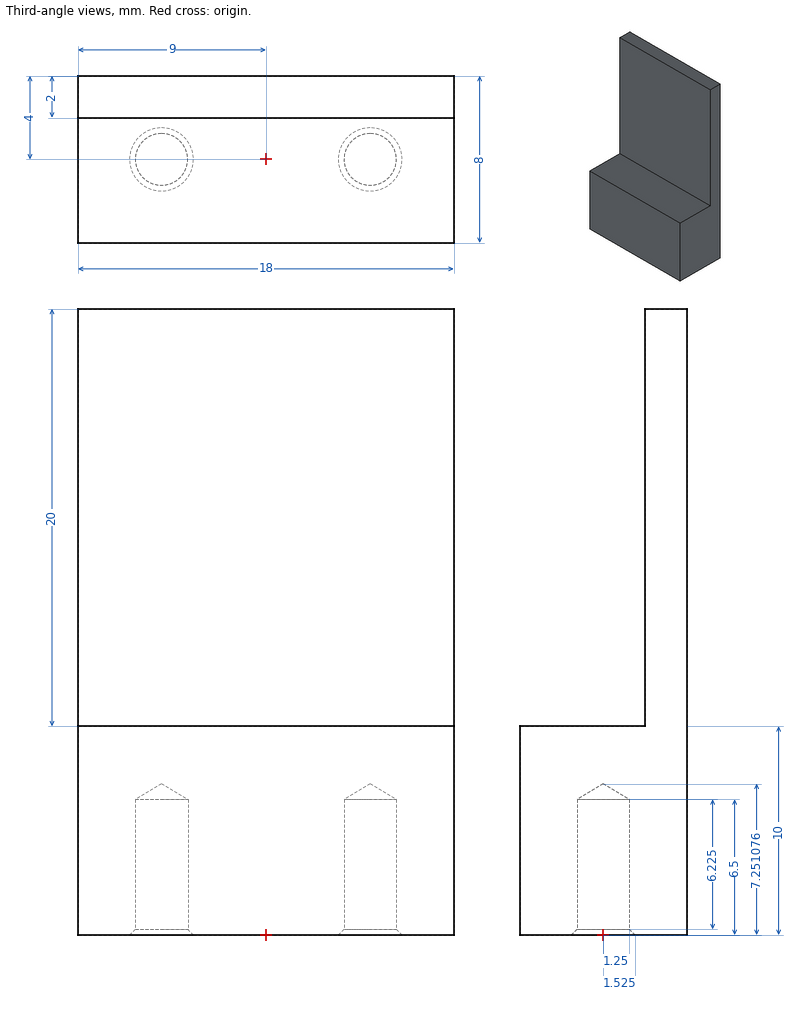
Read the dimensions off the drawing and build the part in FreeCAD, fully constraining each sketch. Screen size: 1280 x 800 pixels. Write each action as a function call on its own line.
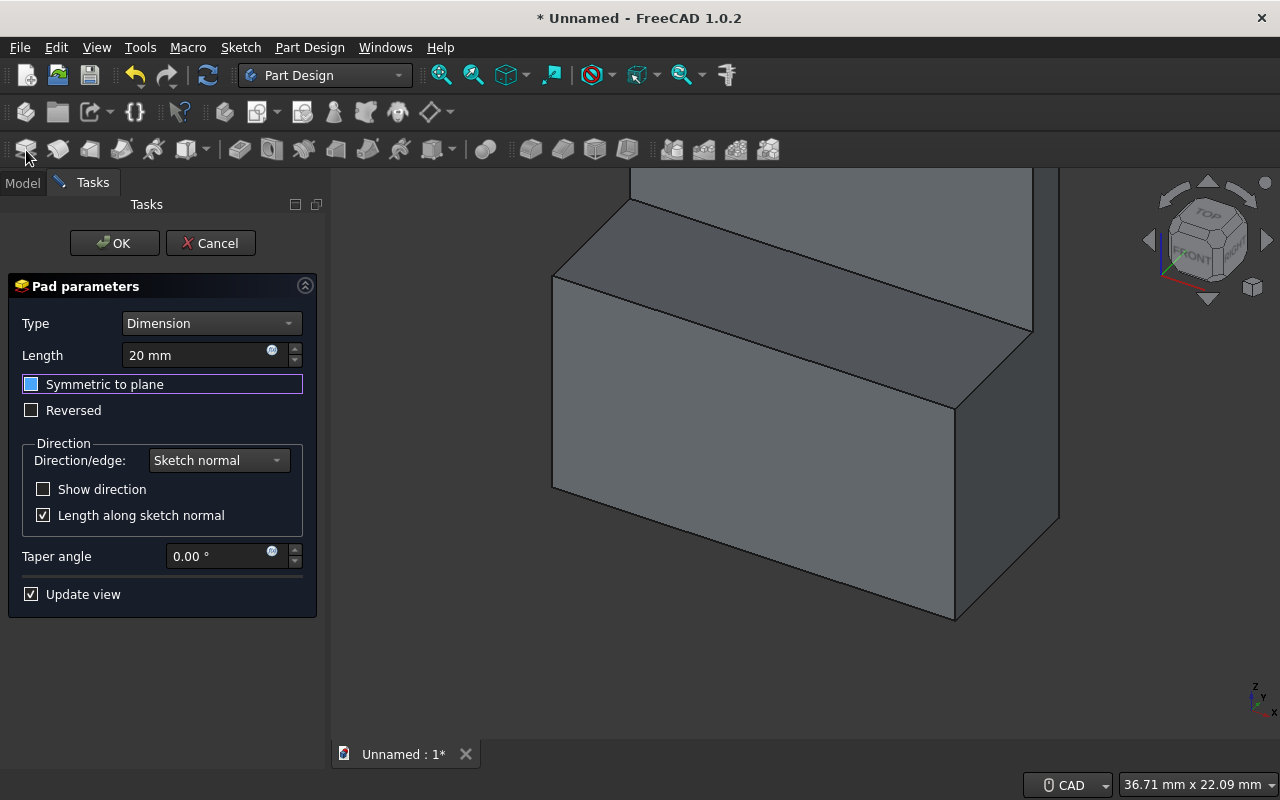
click(115, 243)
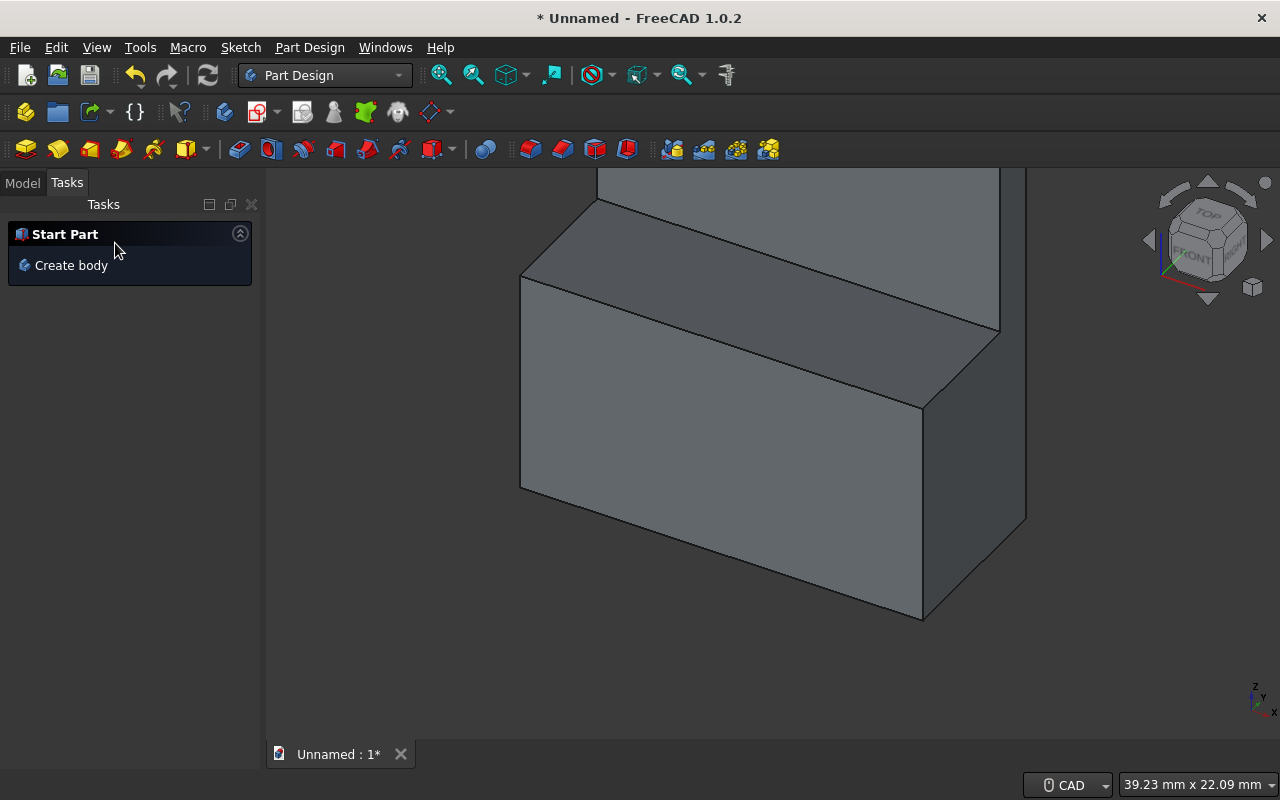
click(442, 76)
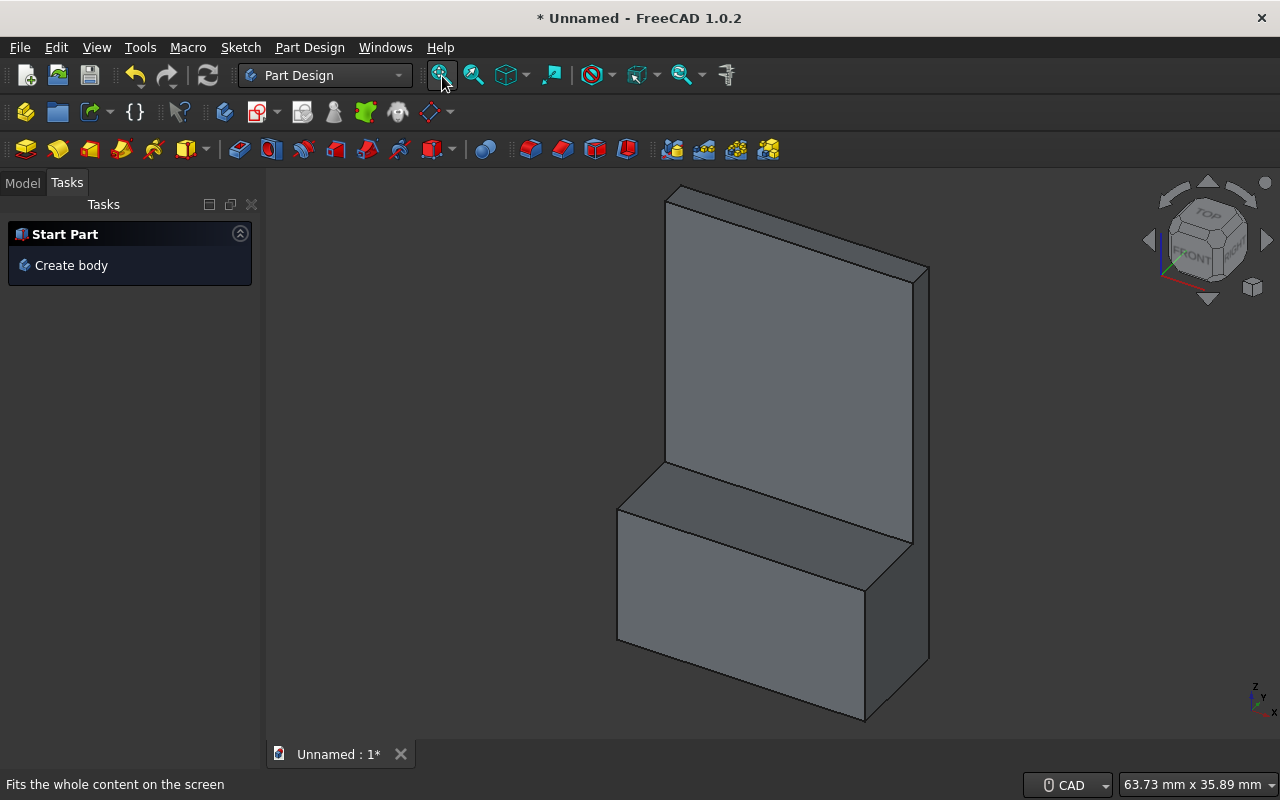
click(23, 182)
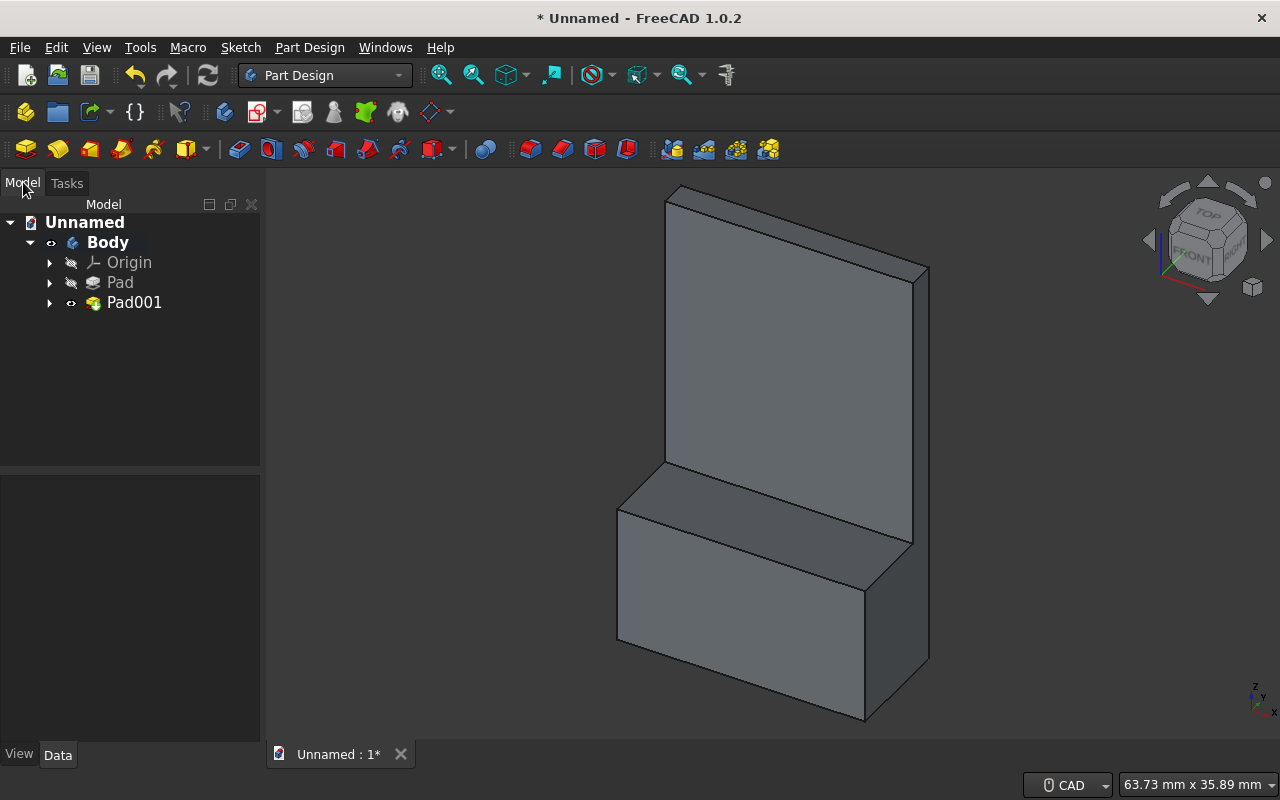
click(50, 263)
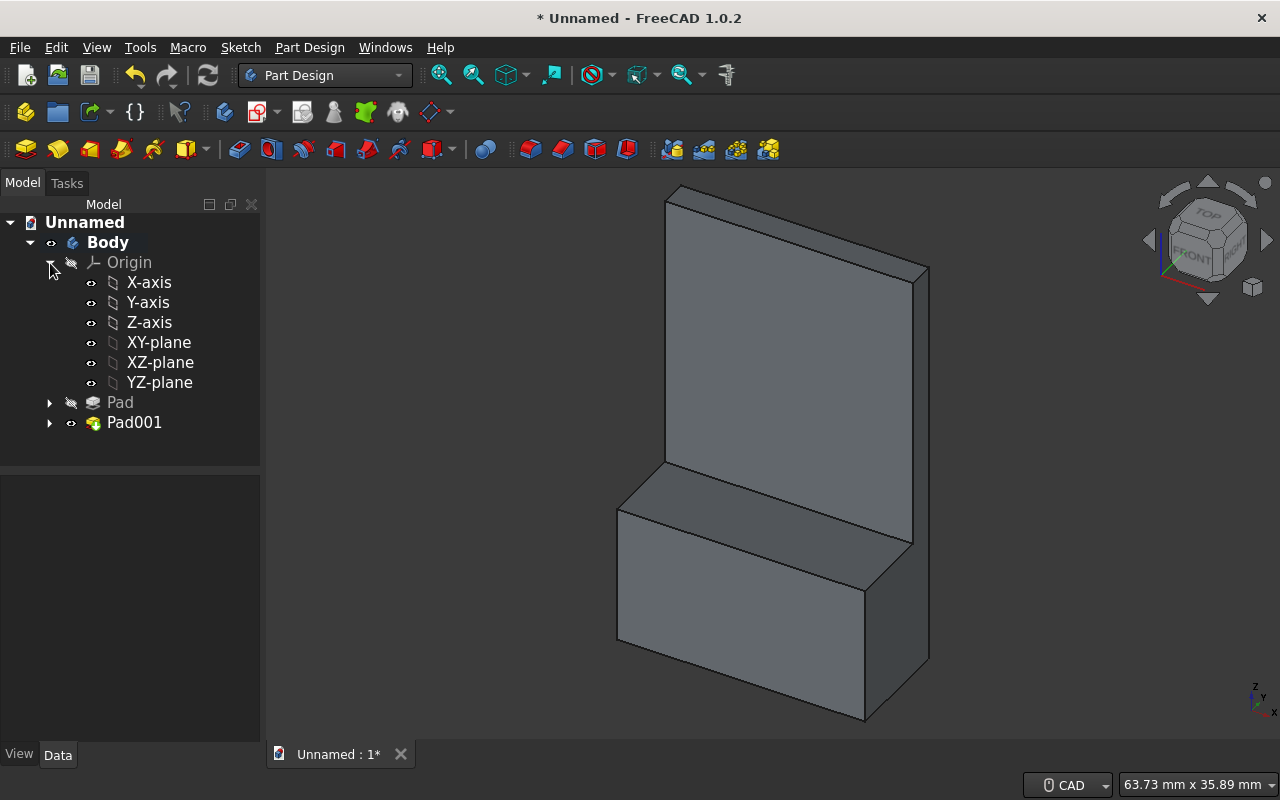
click(136, 383)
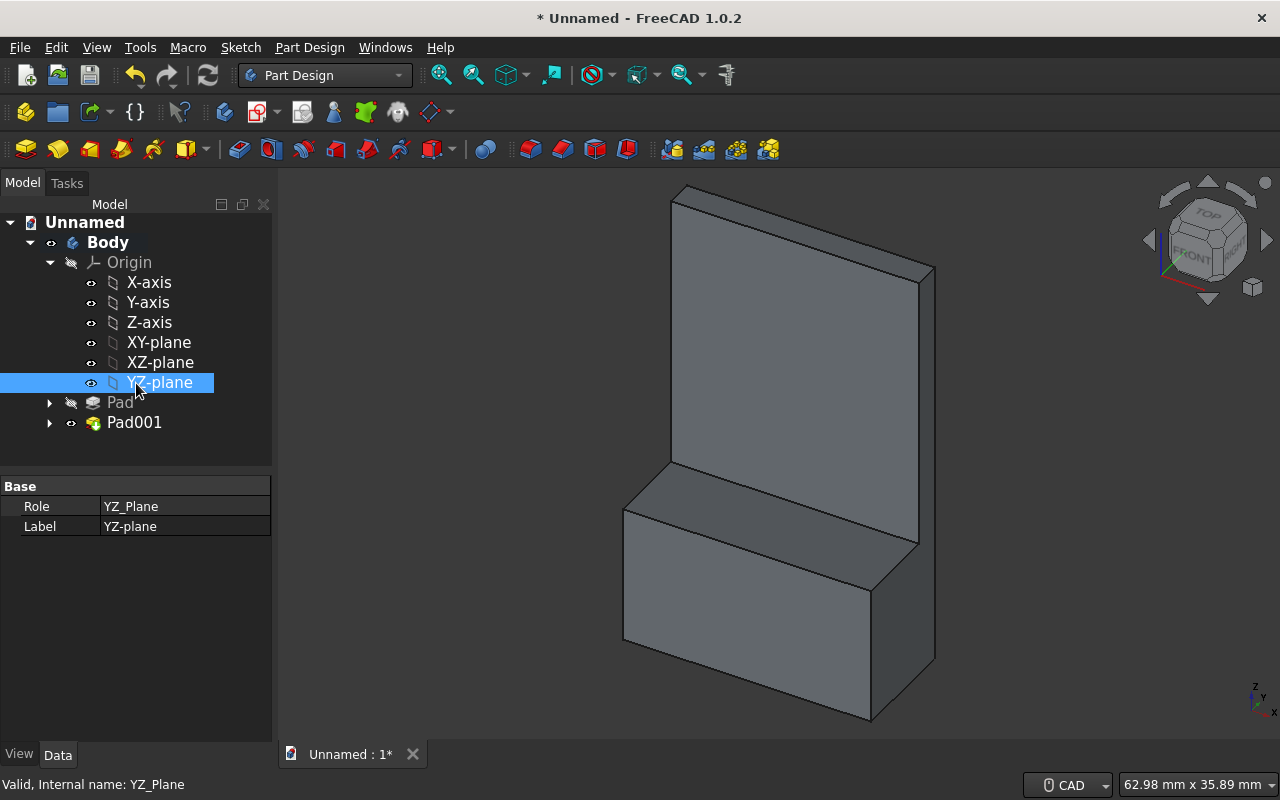
click(430, 112)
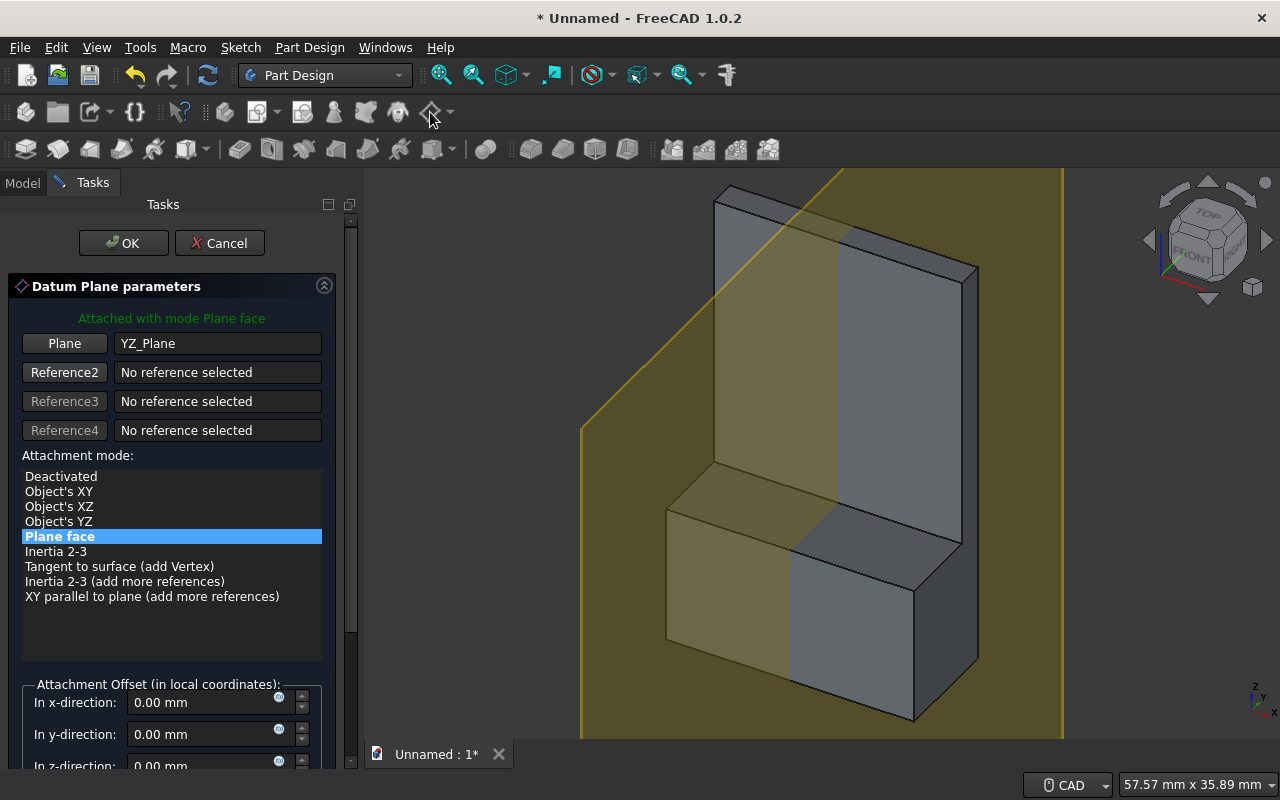
scroll(351, 491, down, 2)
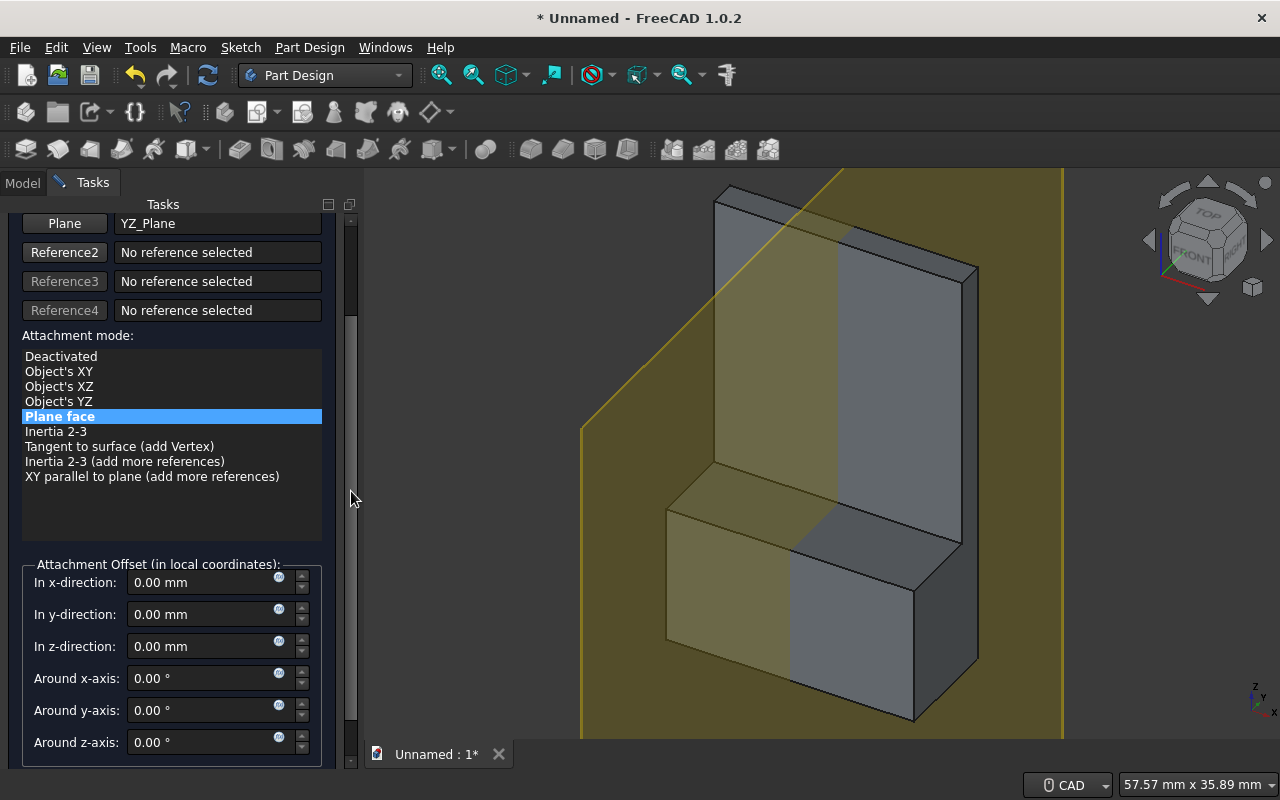
triple_click(210, 646)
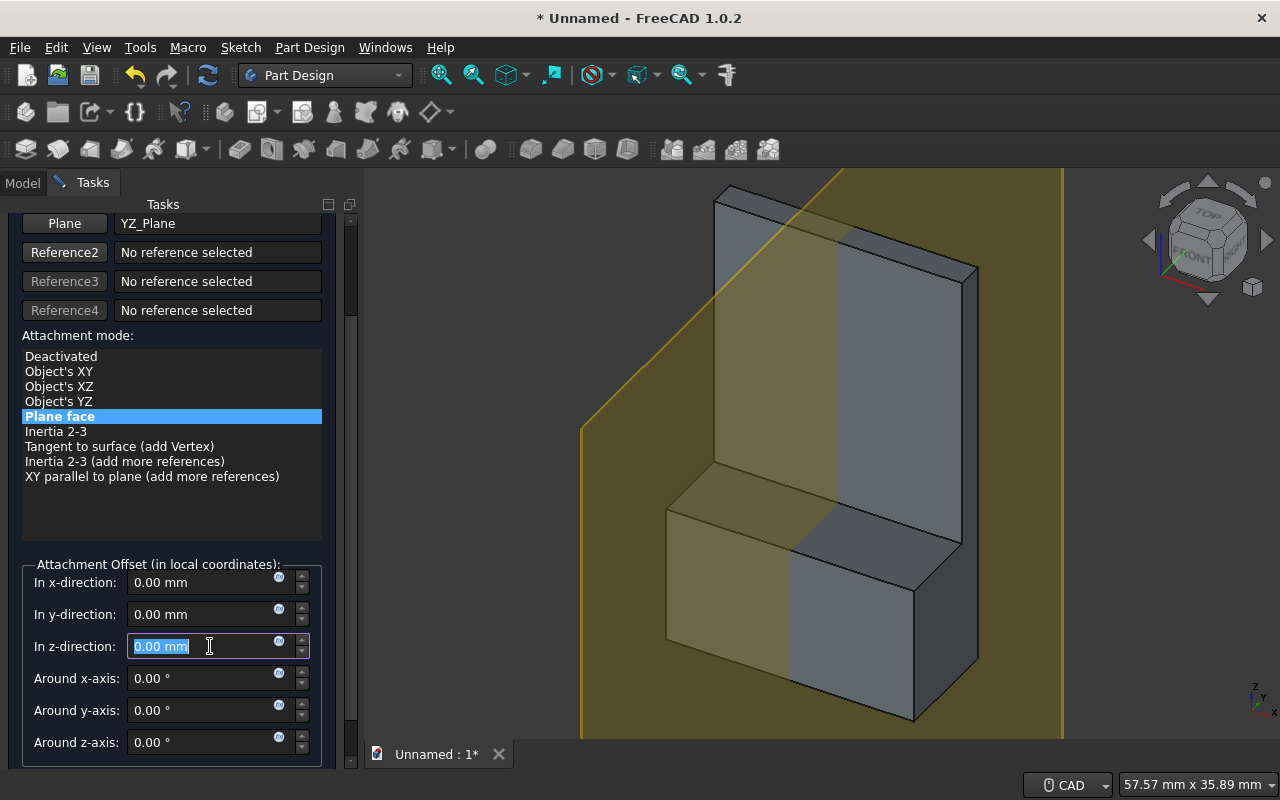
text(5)
key(Tab)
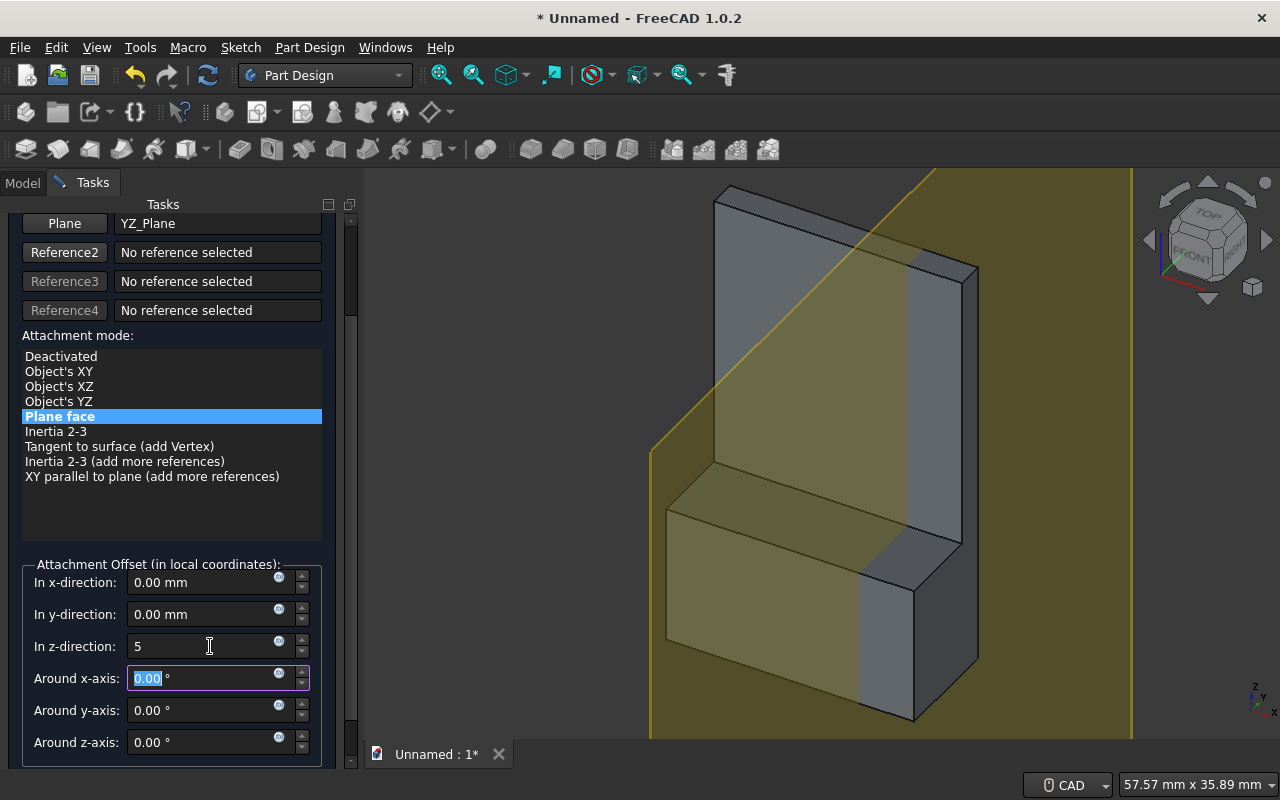
scroll(351, 491, up, 3)